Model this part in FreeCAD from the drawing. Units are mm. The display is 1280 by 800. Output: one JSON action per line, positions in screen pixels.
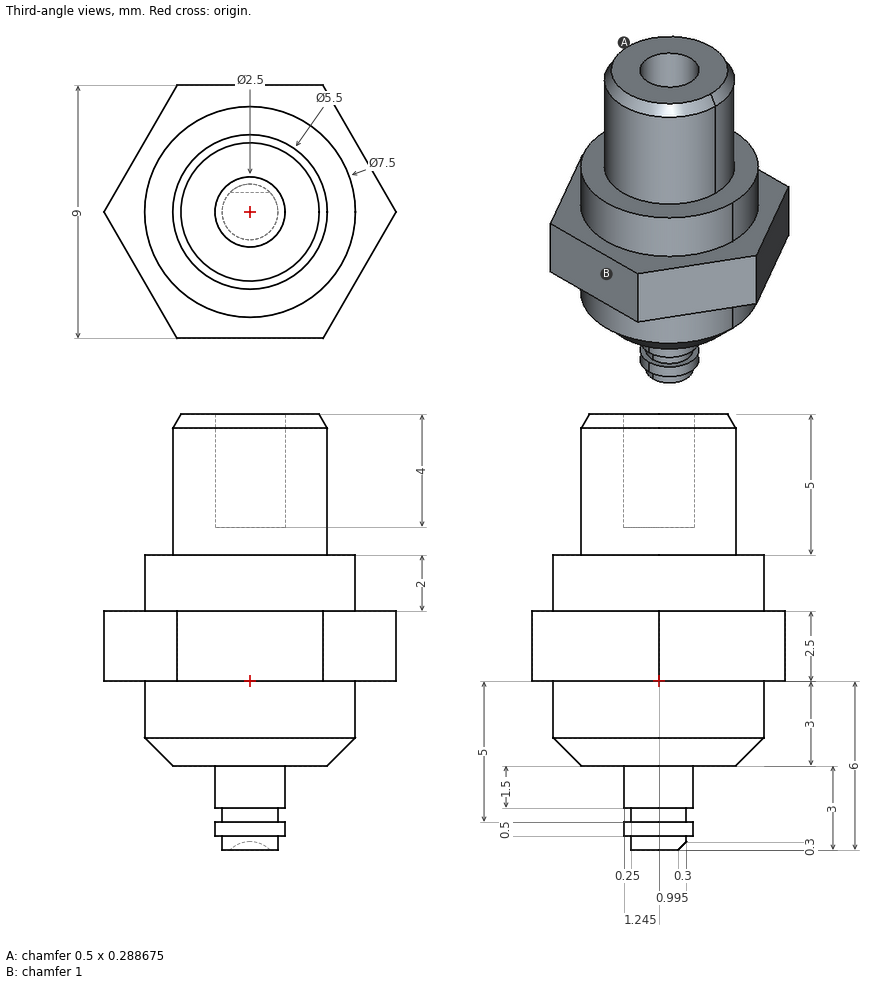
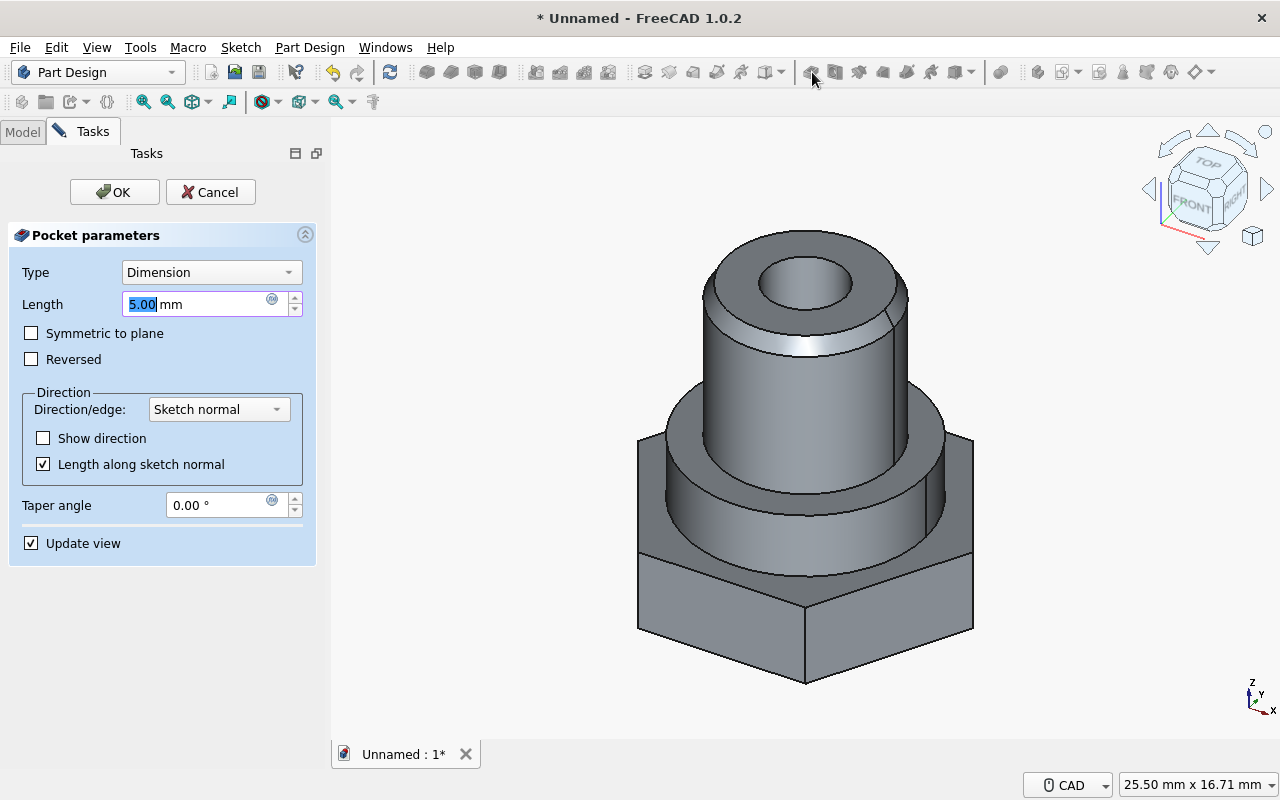
{"action": "type", "text": "4"}
{"action": "key", "text": "Tab"}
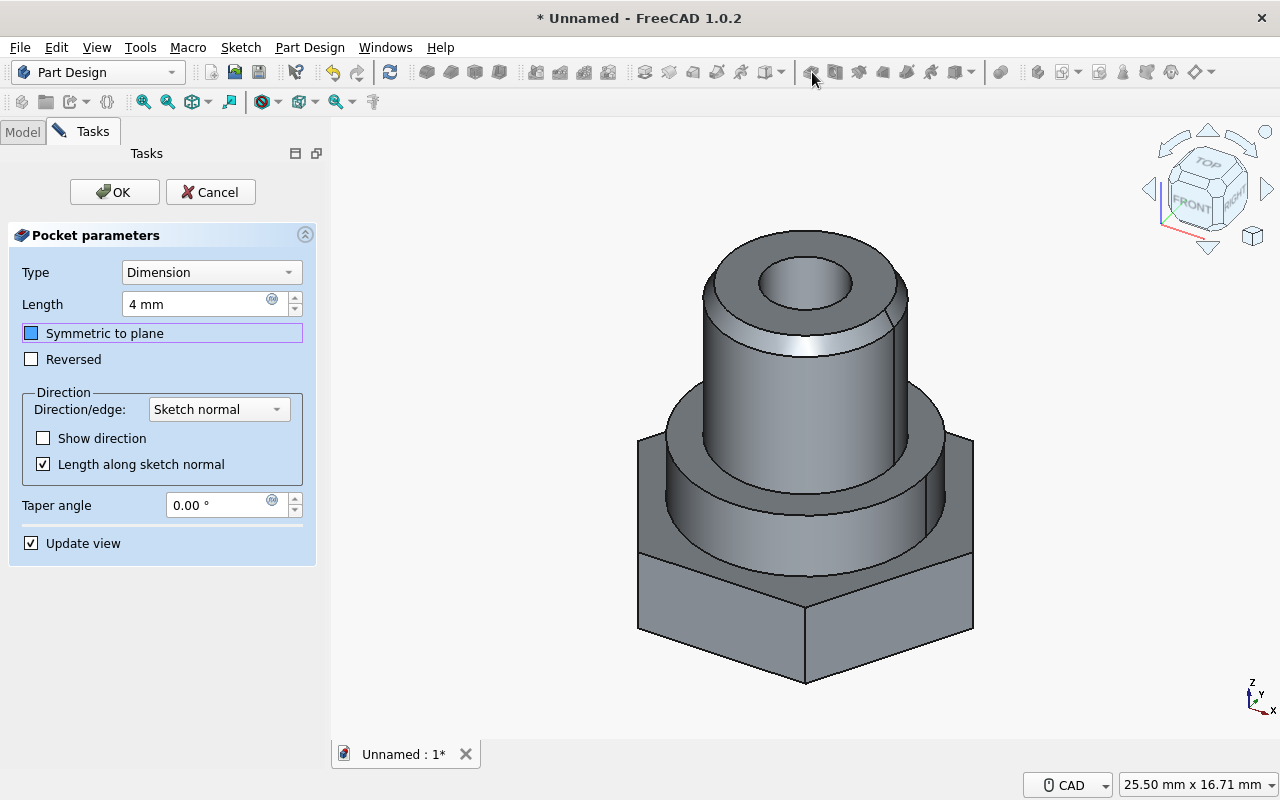
{"action": "left_click", "coordinate": [115, 192]}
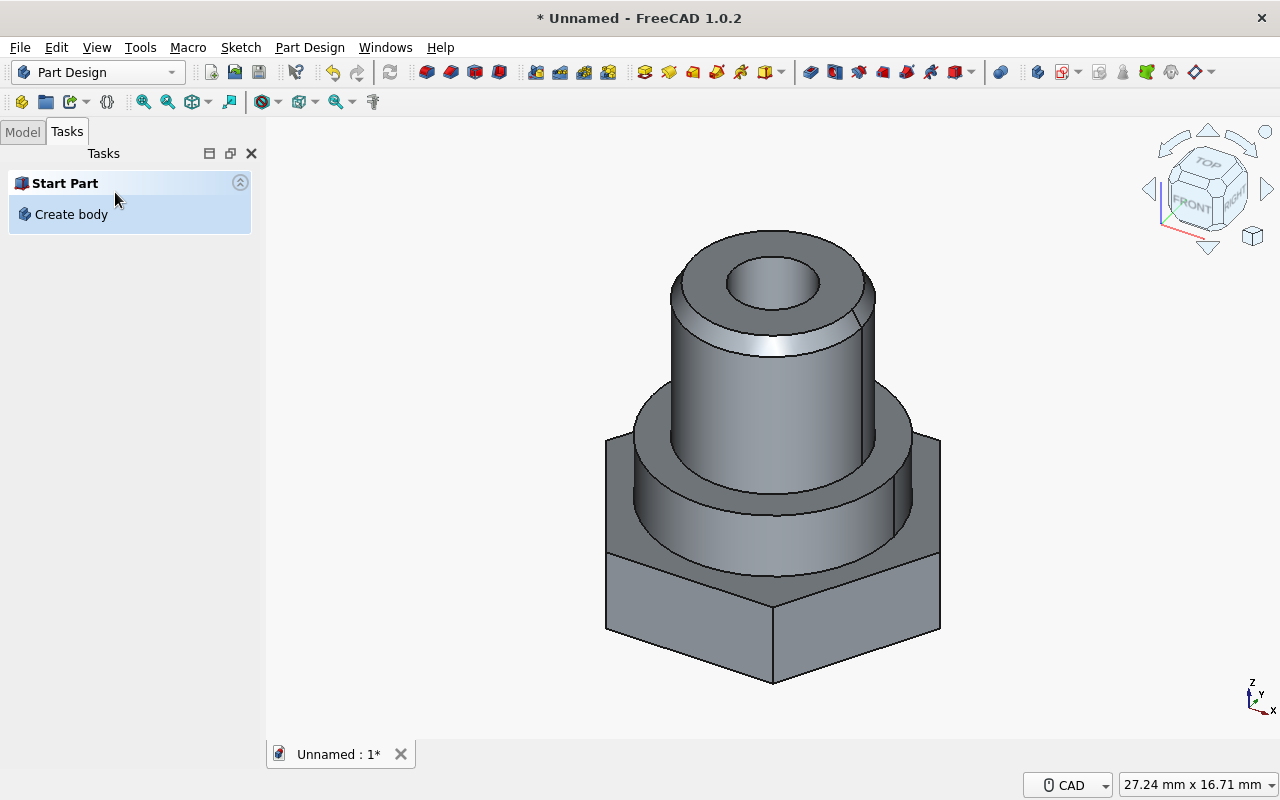
{"action": "left_click", "coordinate": [23, 131]}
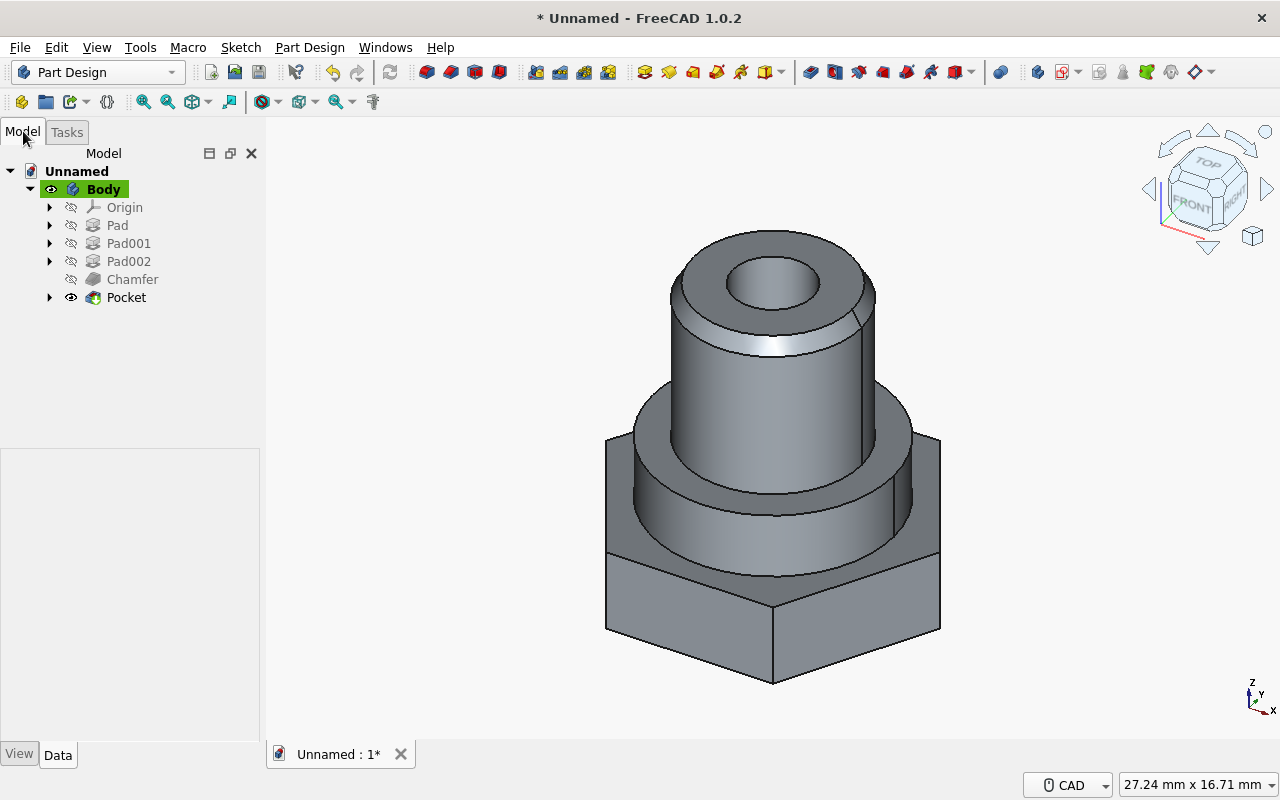
{"action": "left_click", "coordinate": [50, 207]}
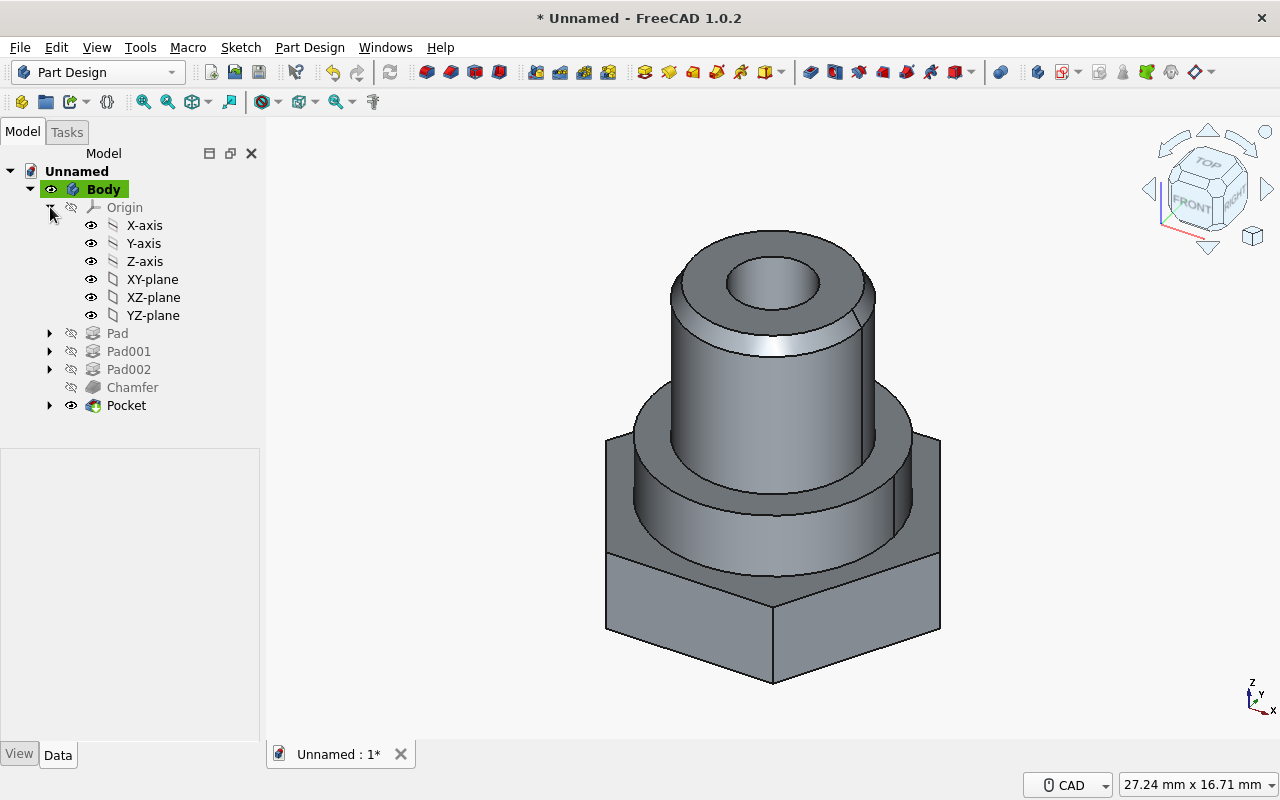
{"action": "left_click", "coordinate": [136, 279]}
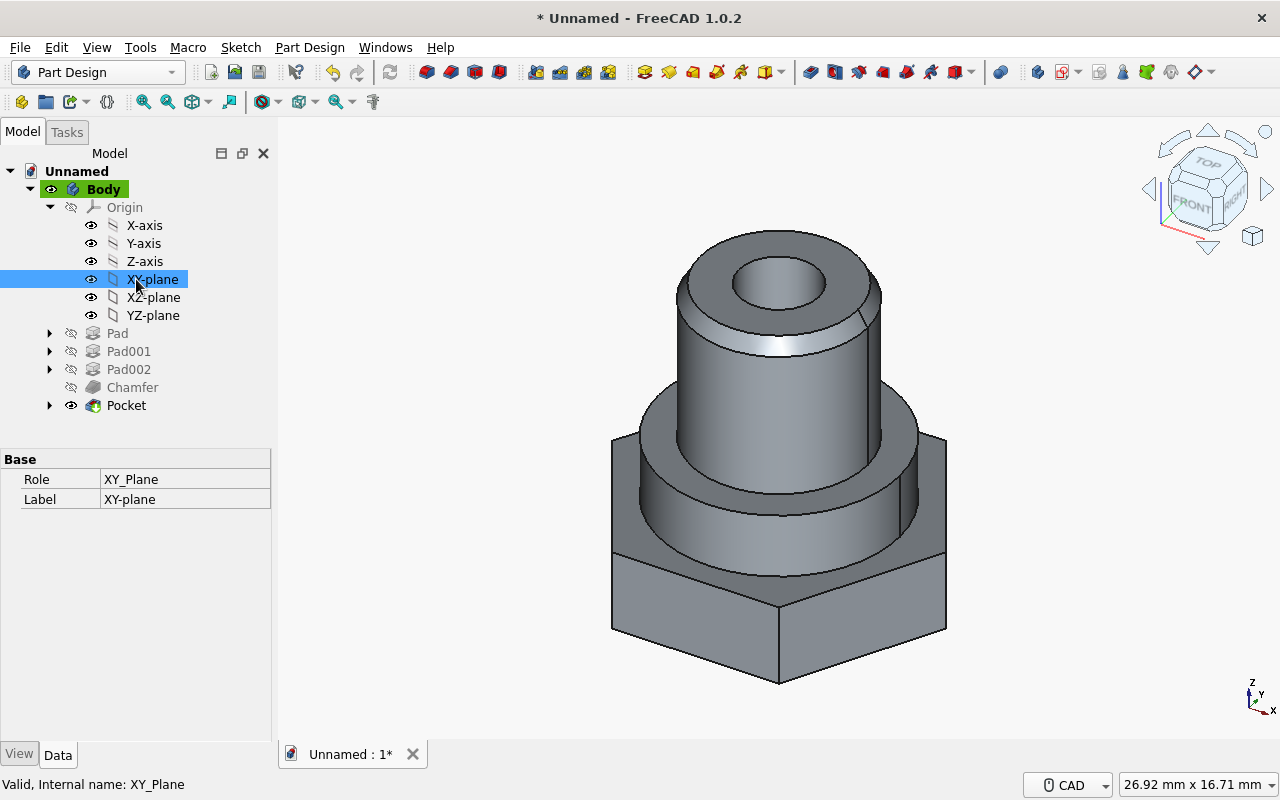
{"action": "left_click", "coordinate": [1196, 72]}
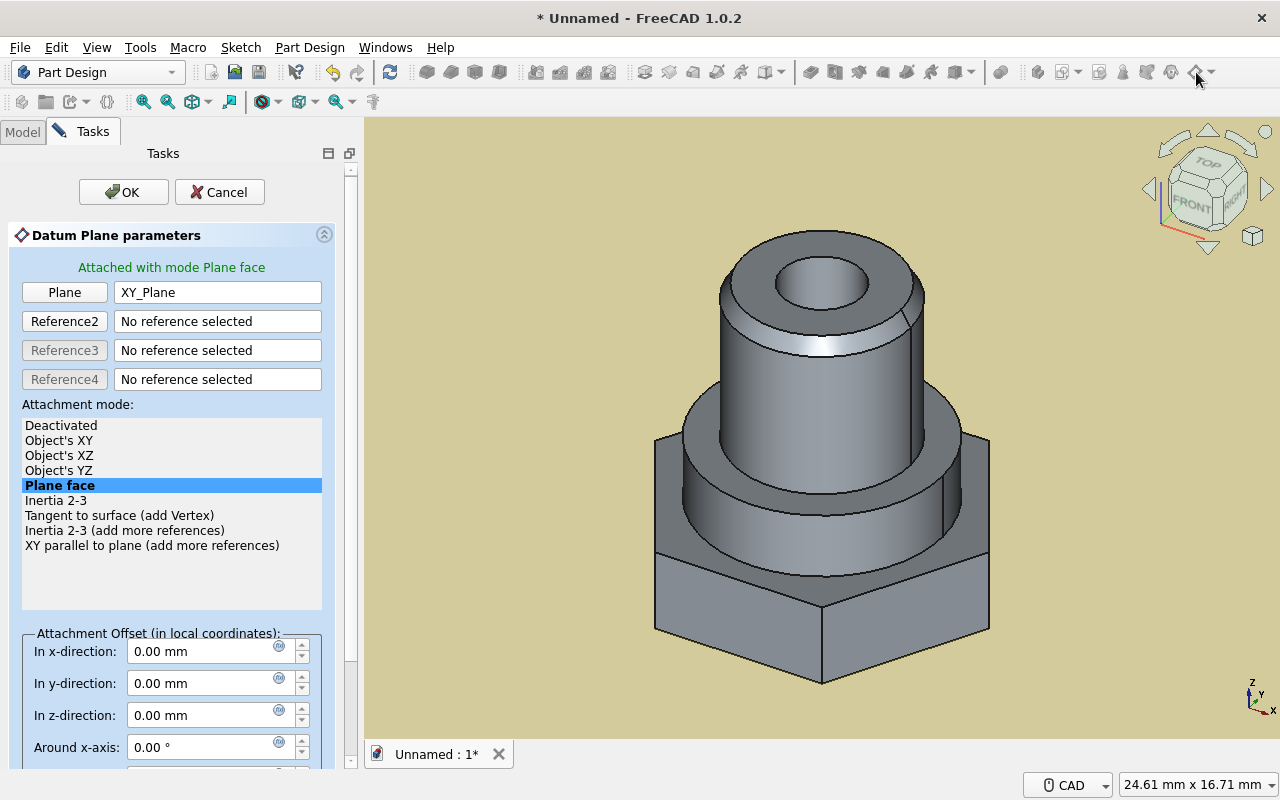
{"action": "triple_click", "coordinate": [210, 715]}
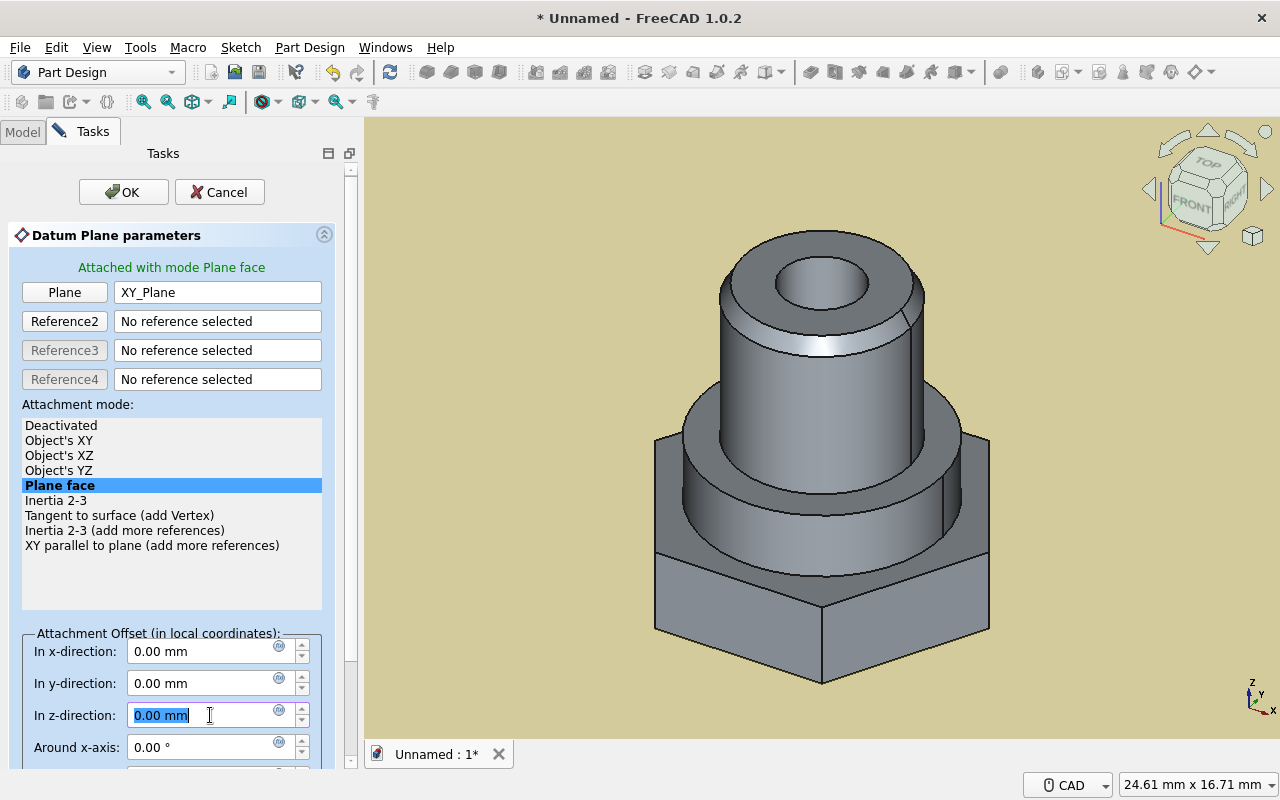
{"action": "type", "text": "-3"}
{"action": "key", "text": "Tab"}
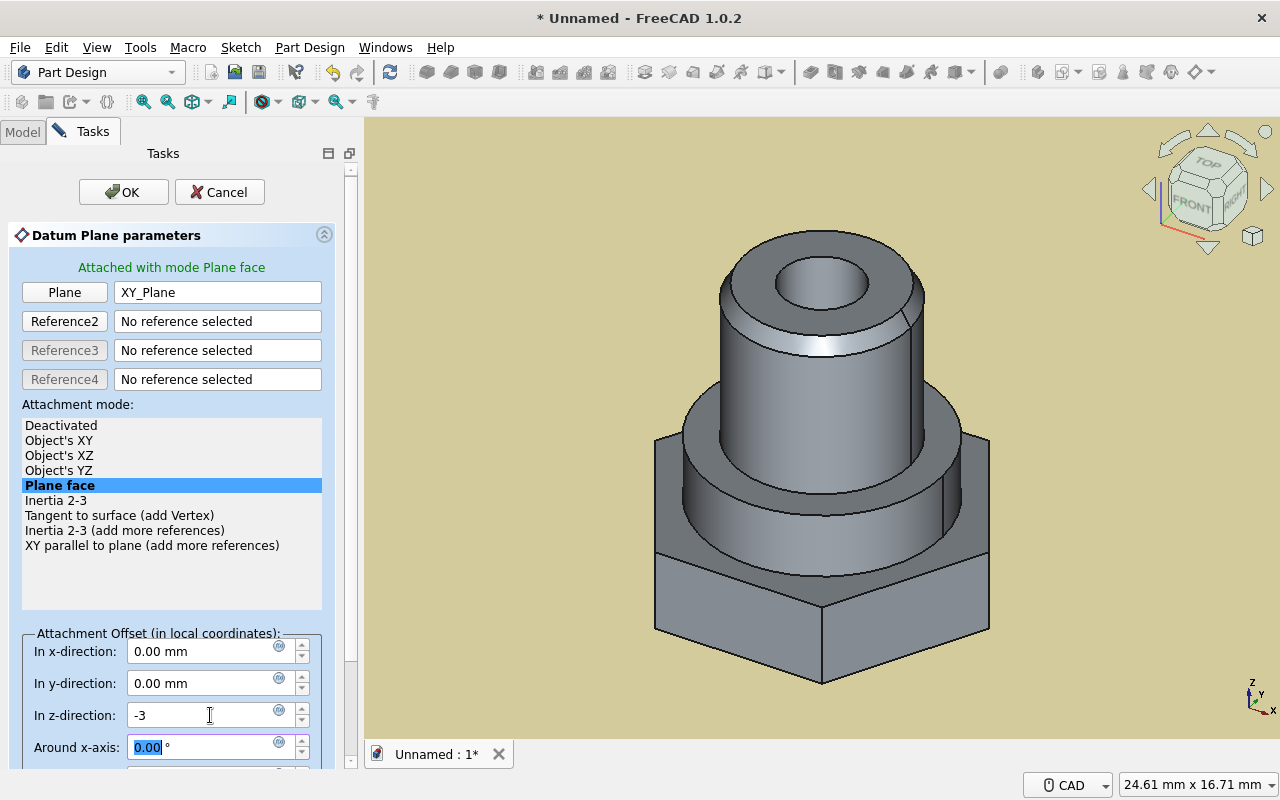
{"action": "left_click", "coordinate": [124, 192]}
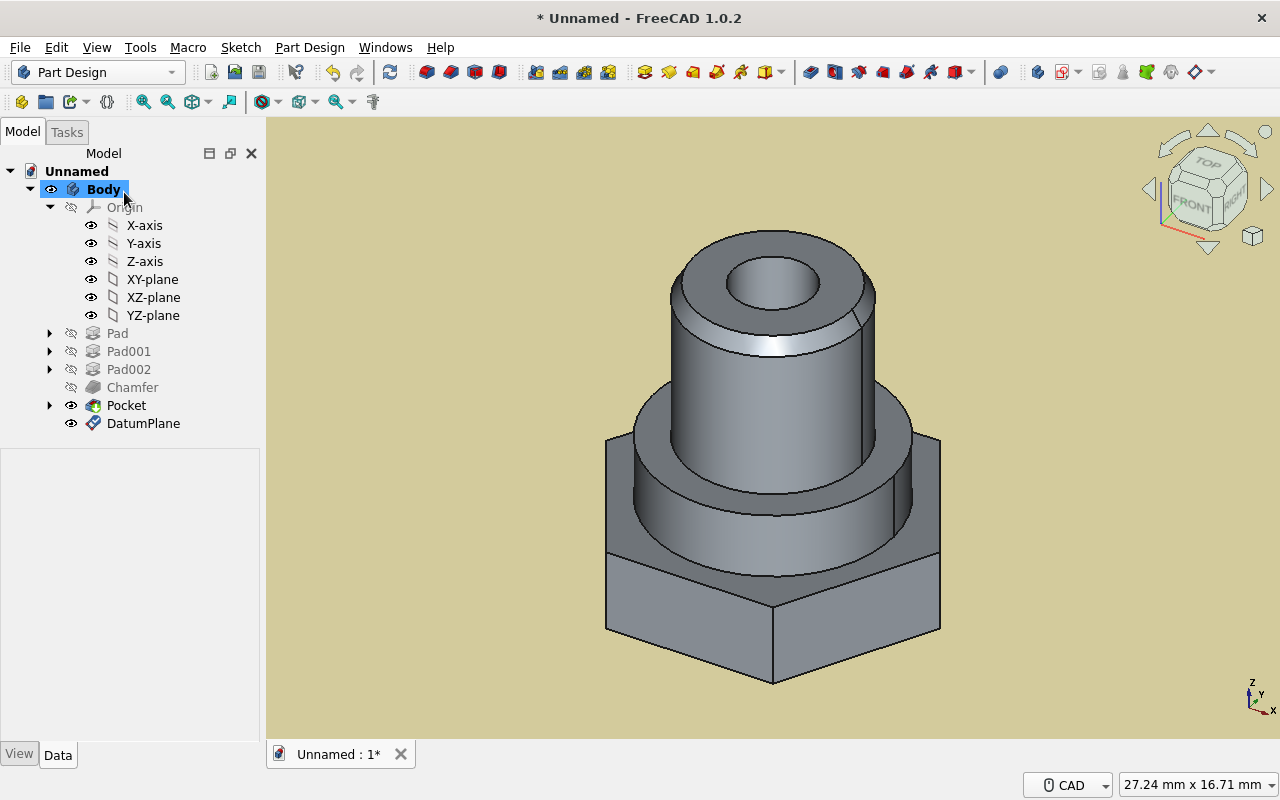
{"action": "left_click", "coordinate": [116, 423]}